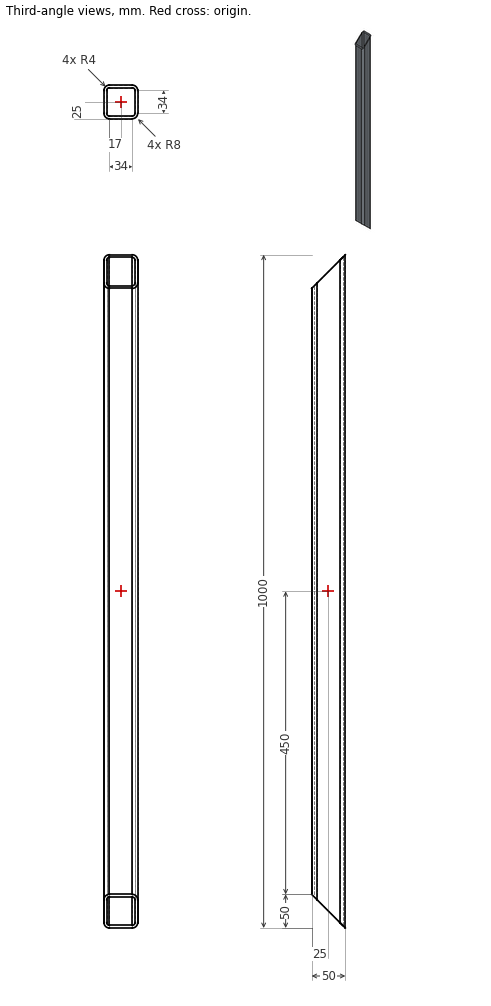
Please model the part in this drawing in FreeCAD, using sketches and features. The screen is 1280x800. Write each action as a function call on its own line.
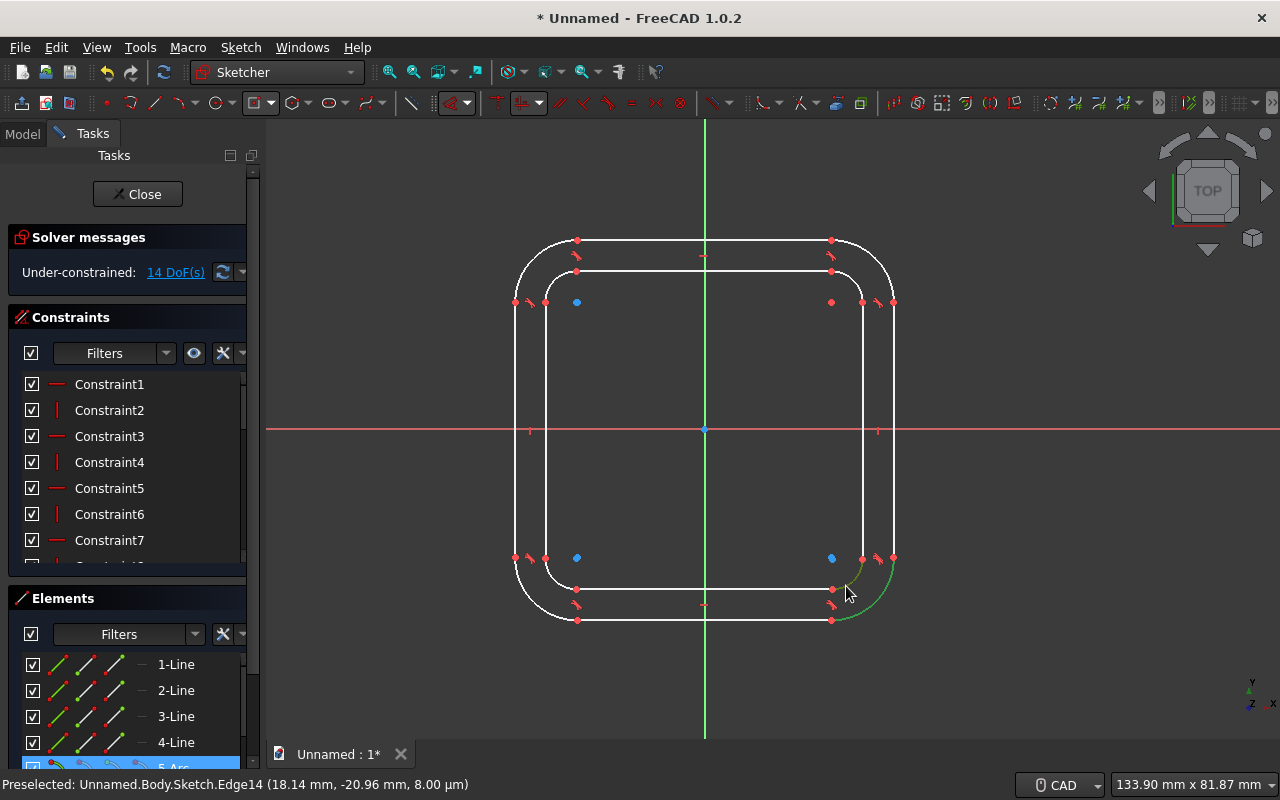
click(498, 104)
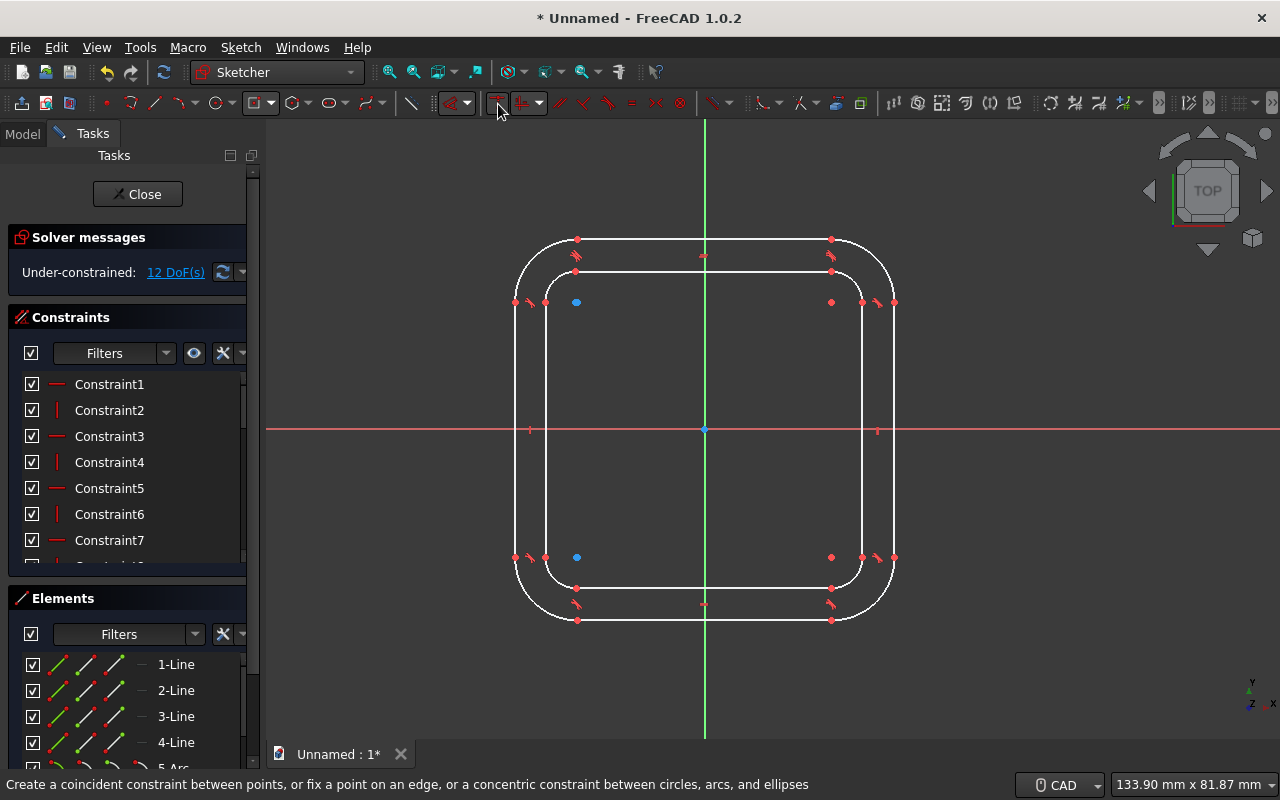
click(522, 586)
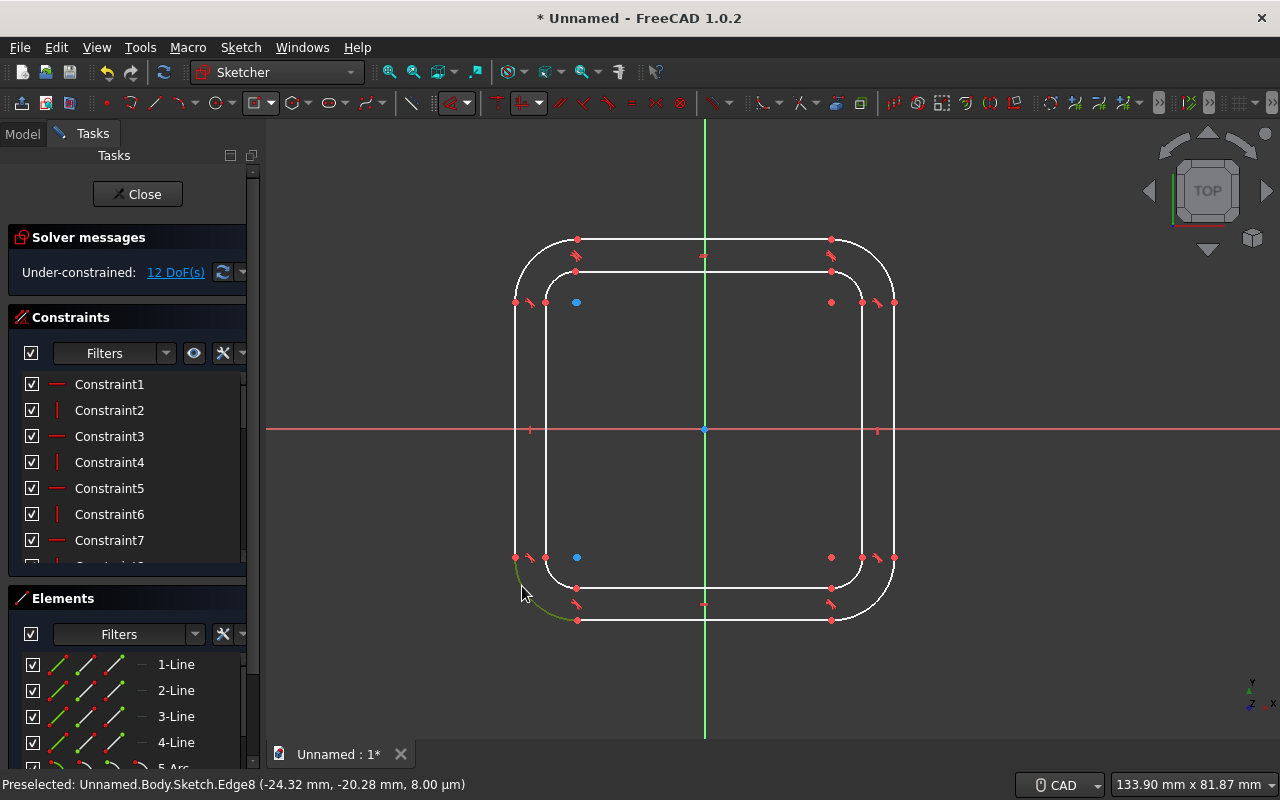
click(549, 571)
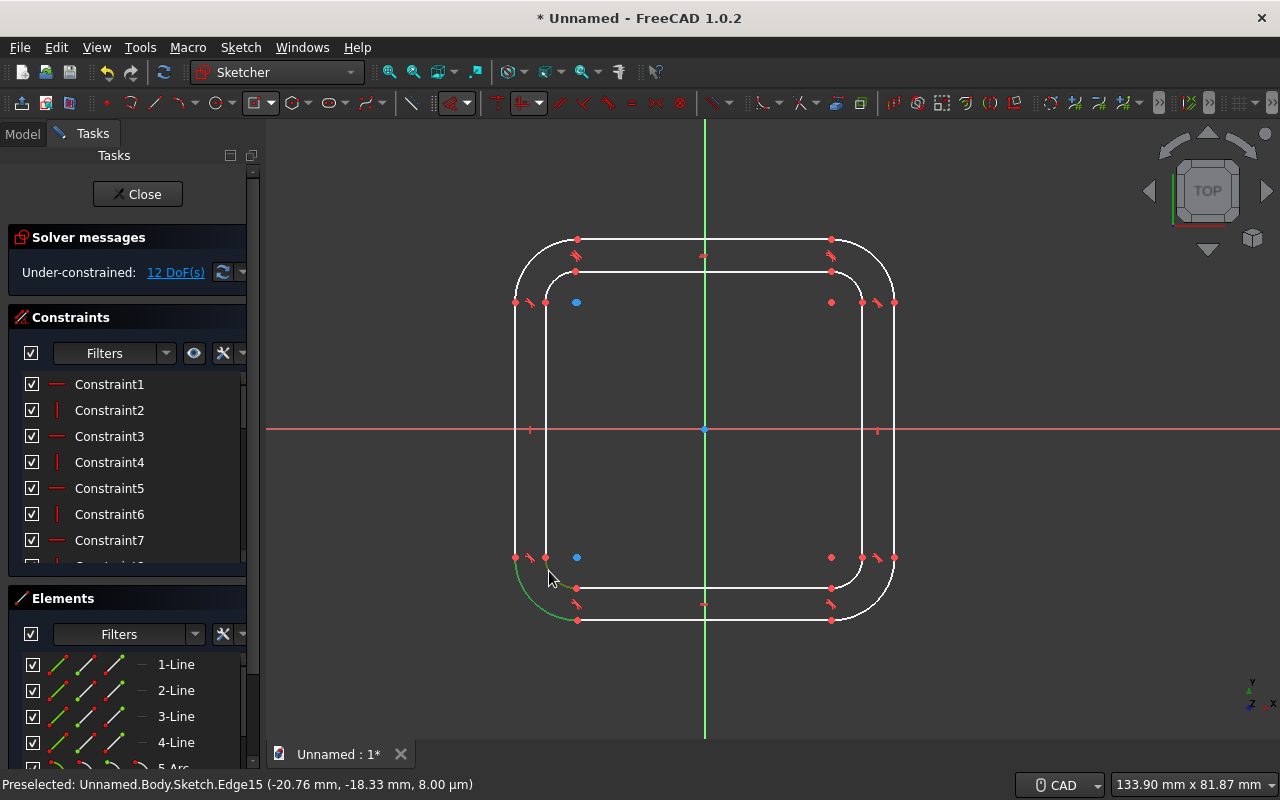
key(c)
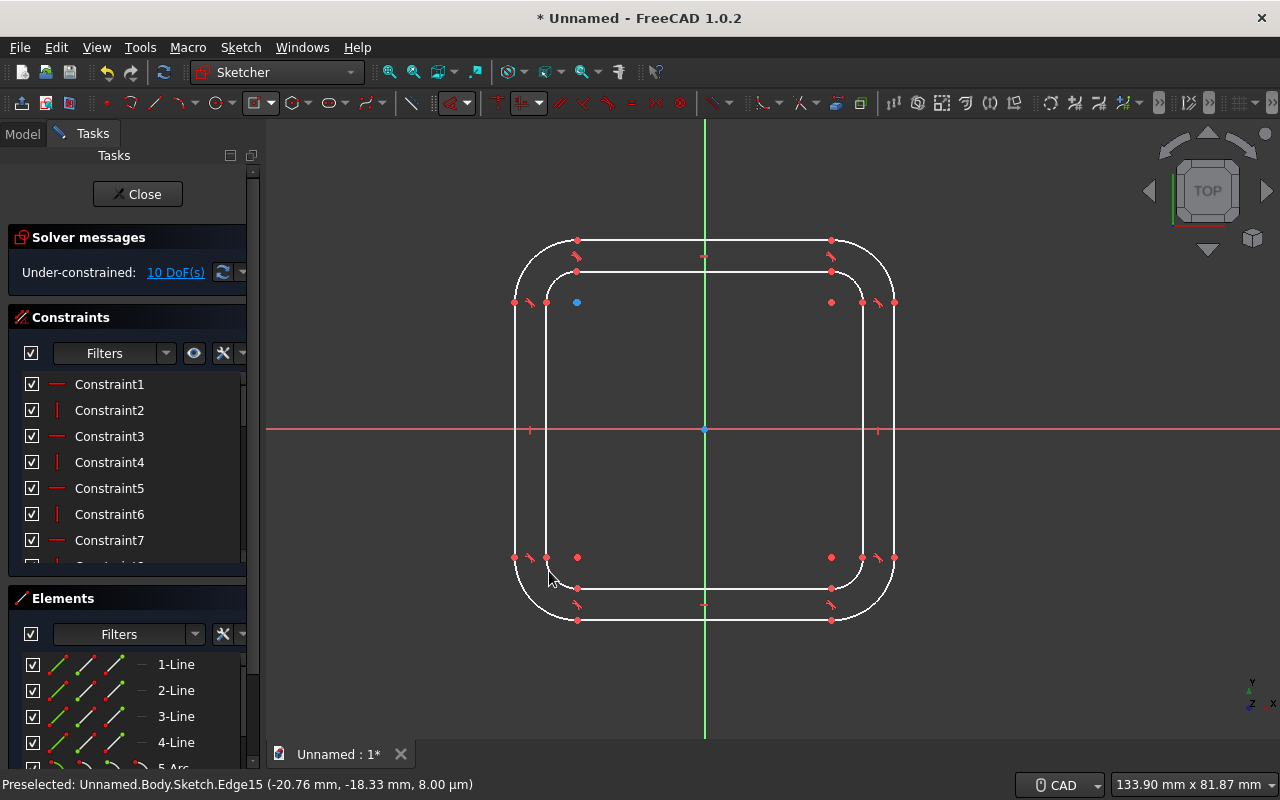
click(860, 614)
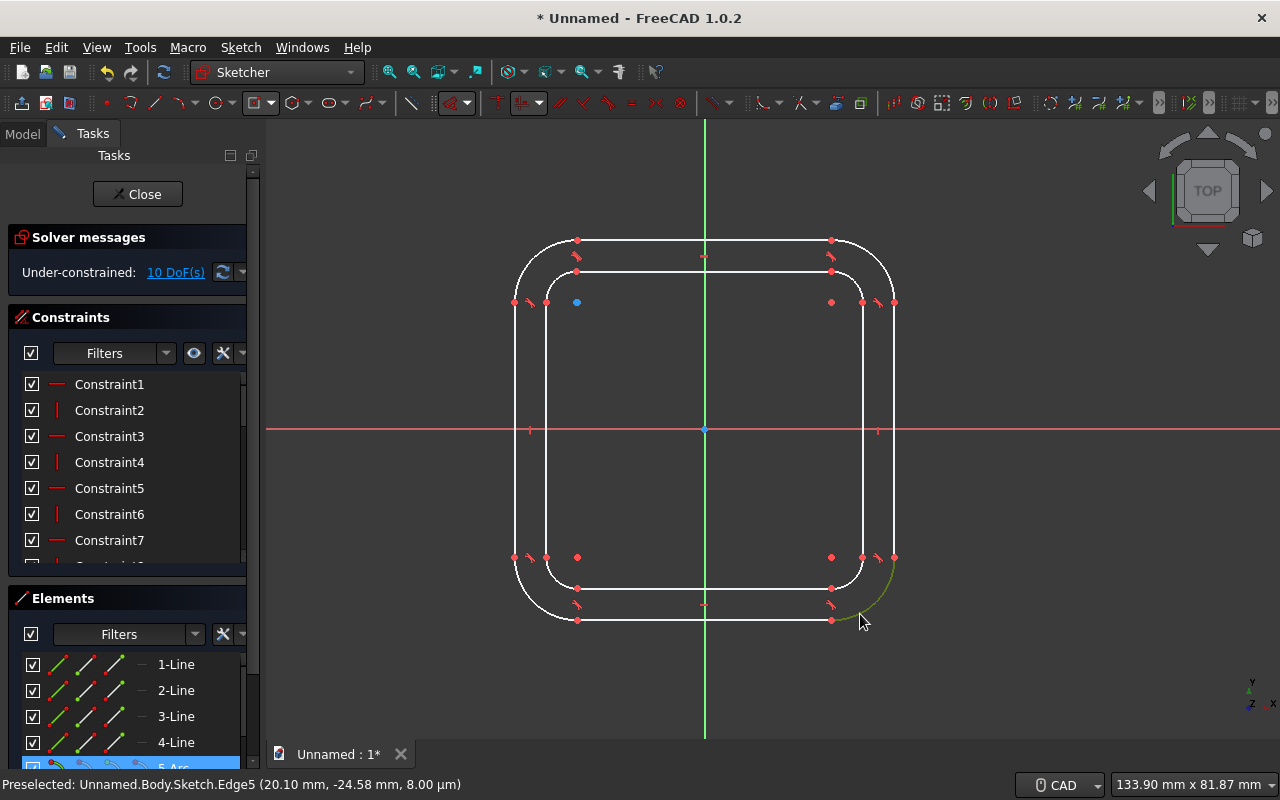
click(888, 274)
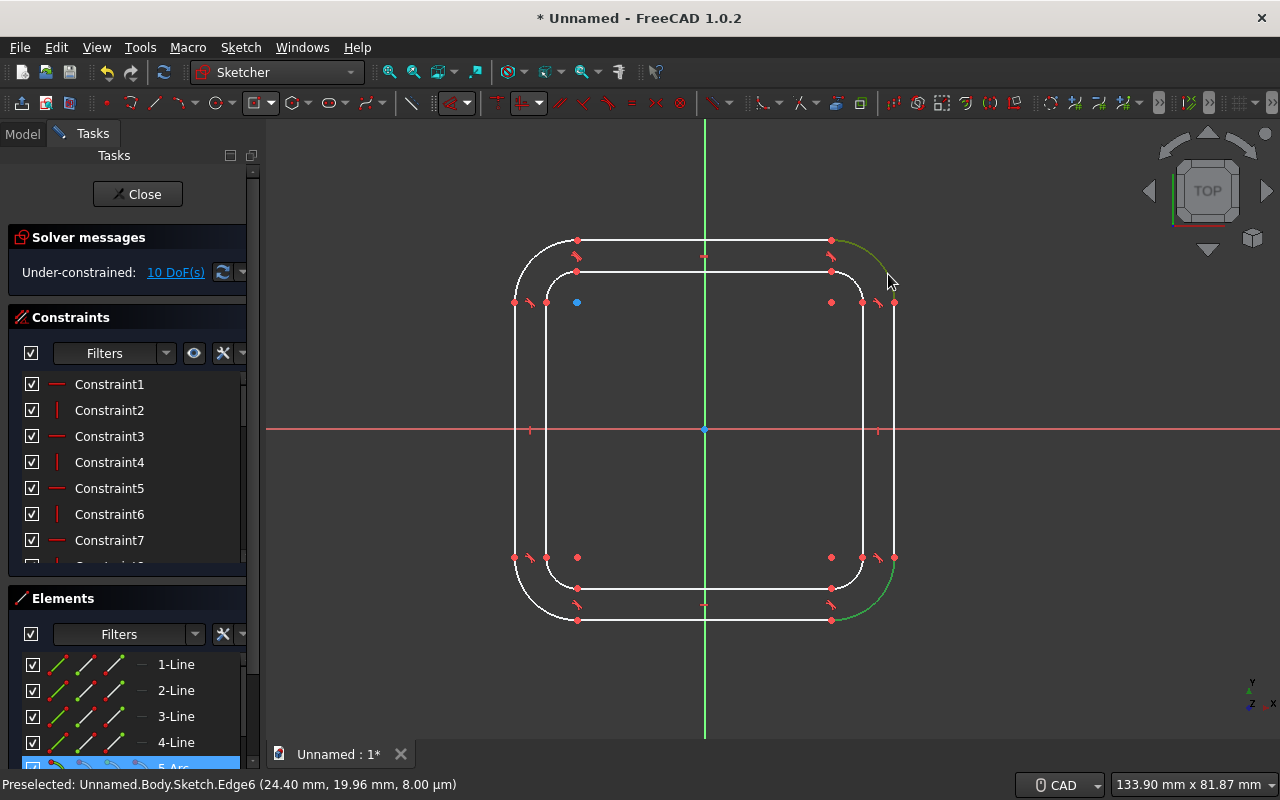
click(549, 247)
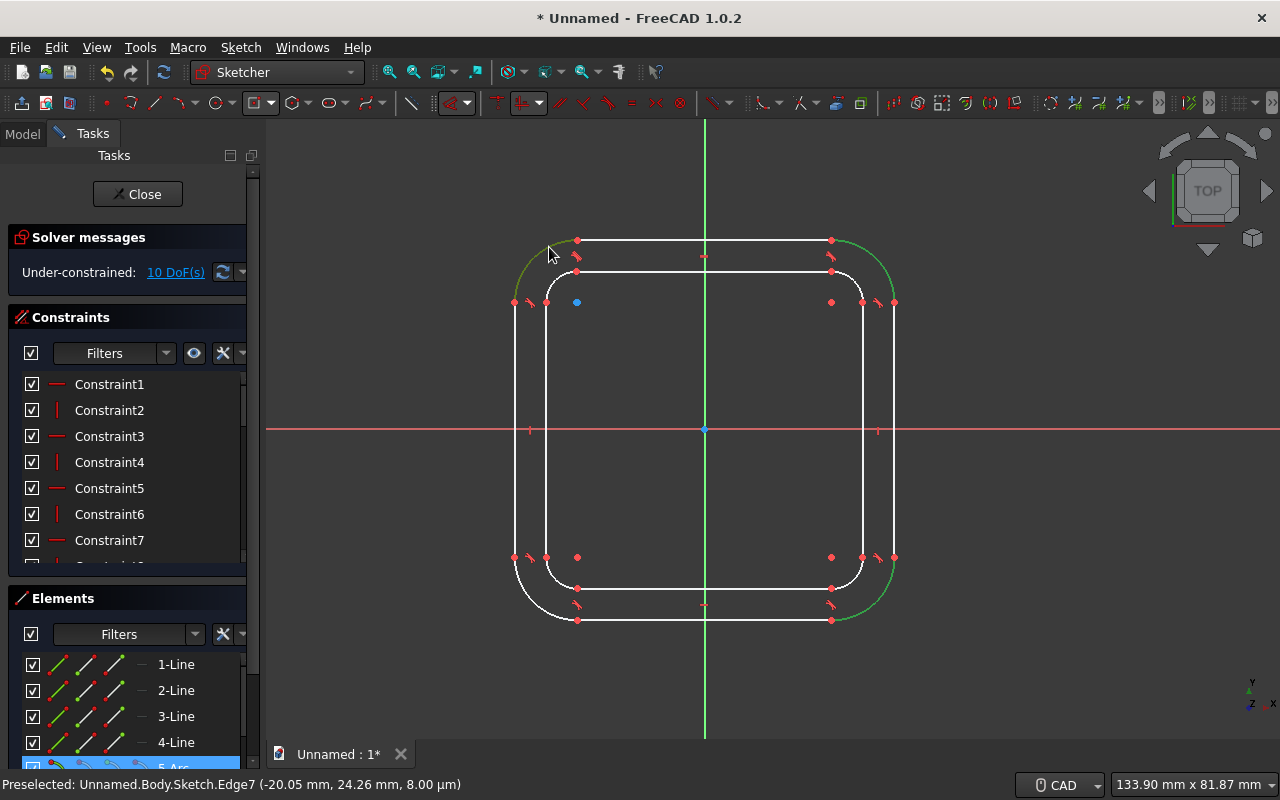
click(522, 586)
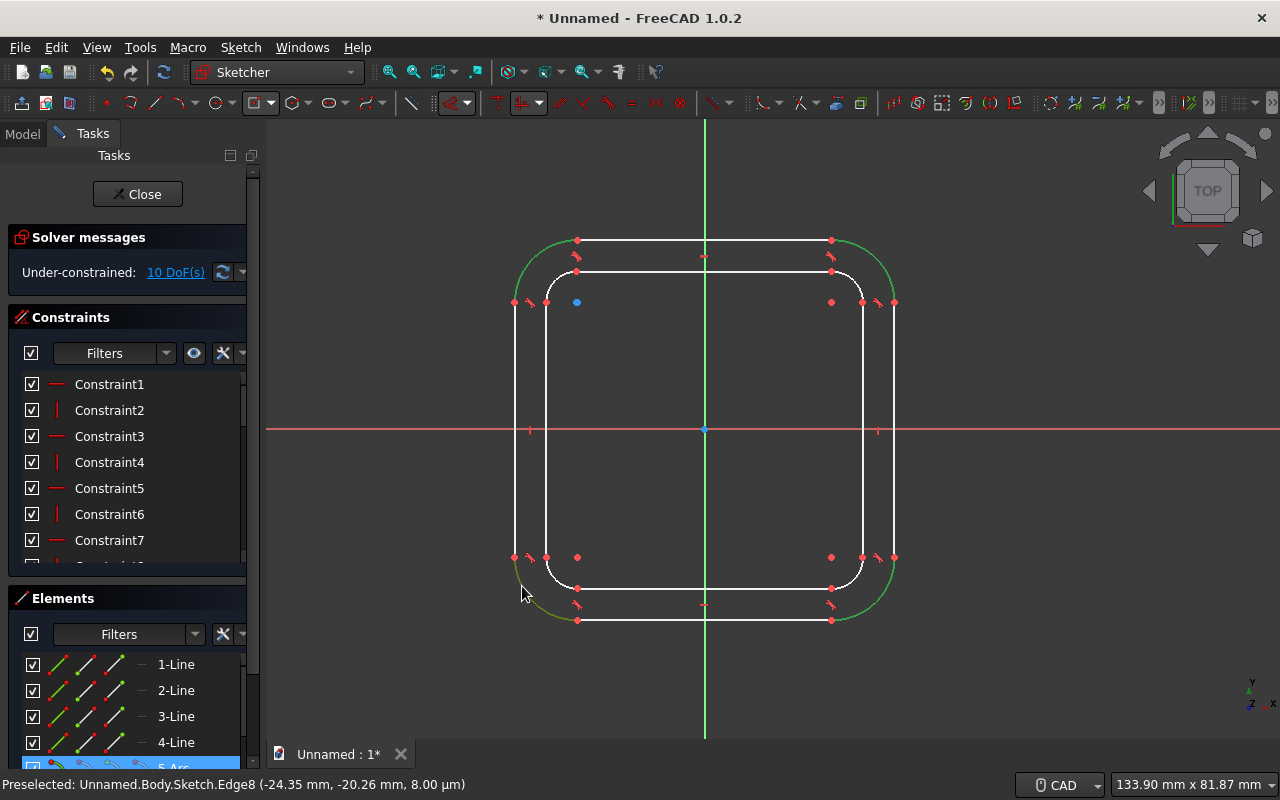
key(e)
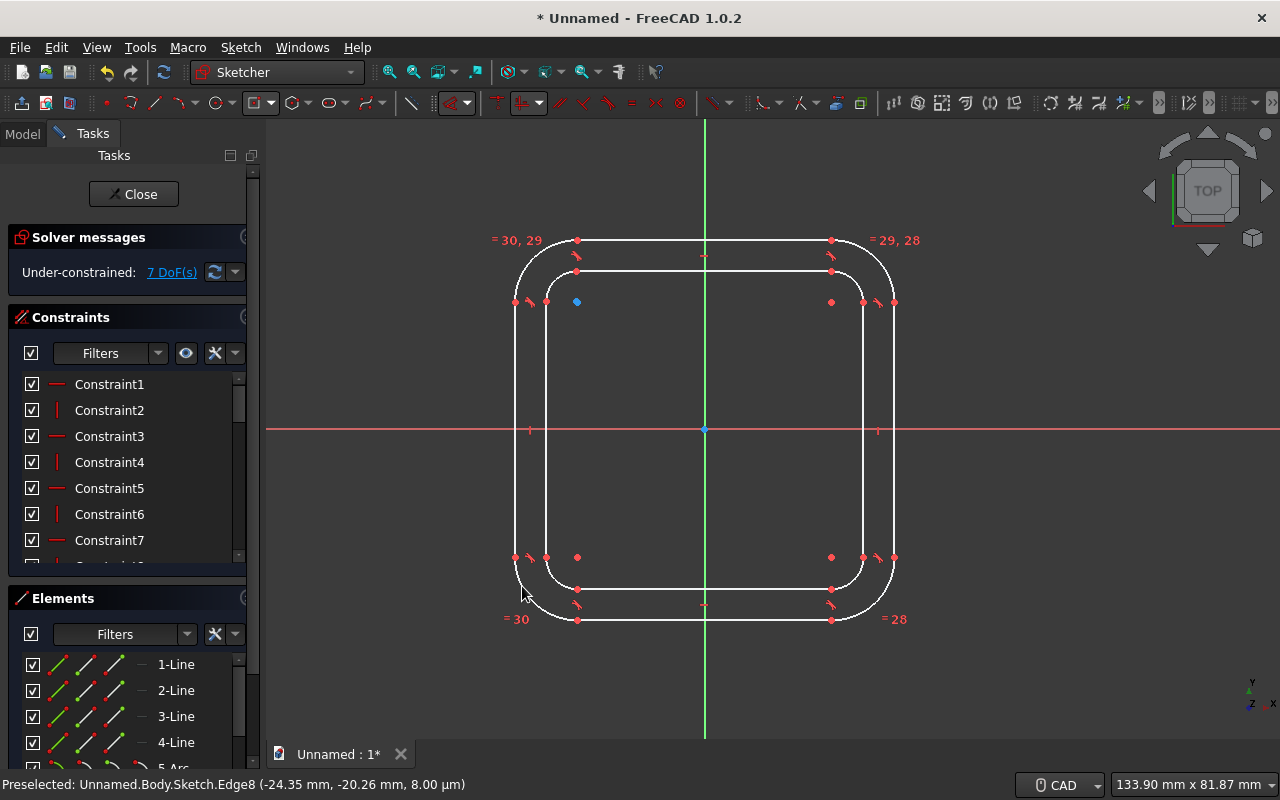
click(860, 288)